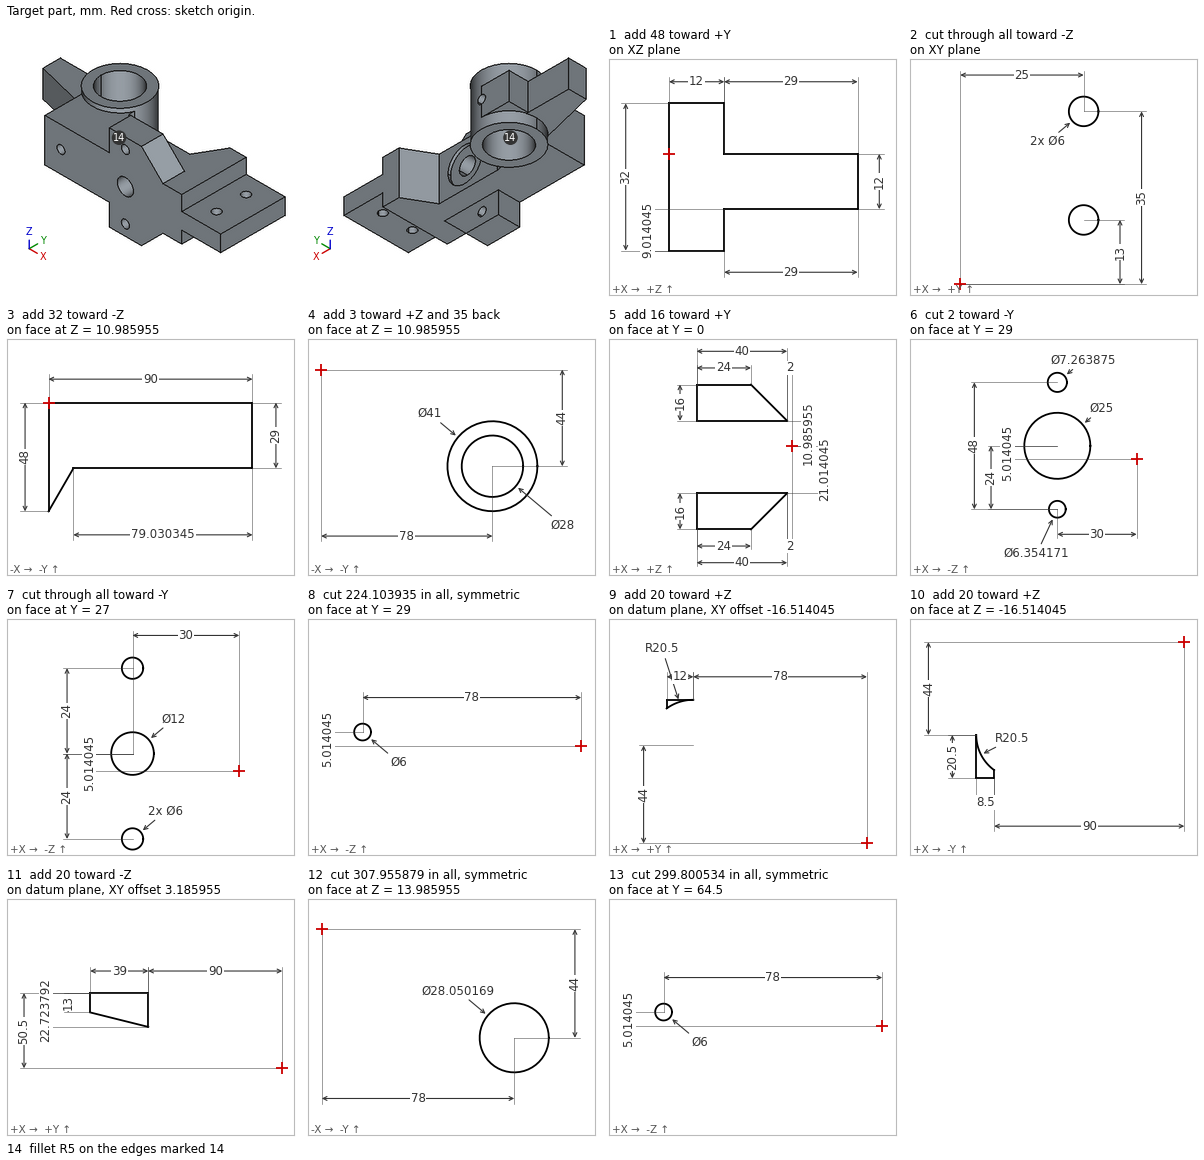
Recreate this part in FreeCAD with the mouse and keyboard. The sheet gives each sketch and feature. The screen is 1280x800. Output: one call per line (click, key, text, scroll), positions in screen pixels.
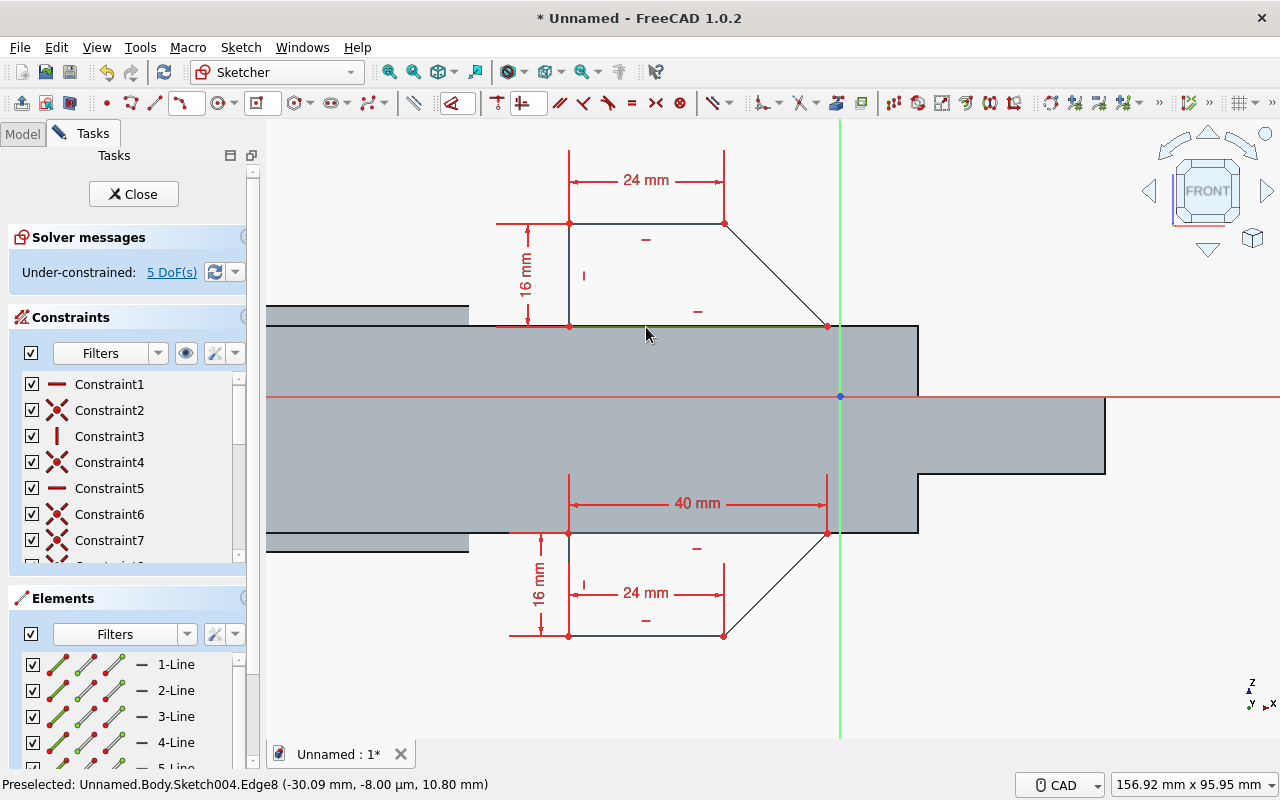
key(l)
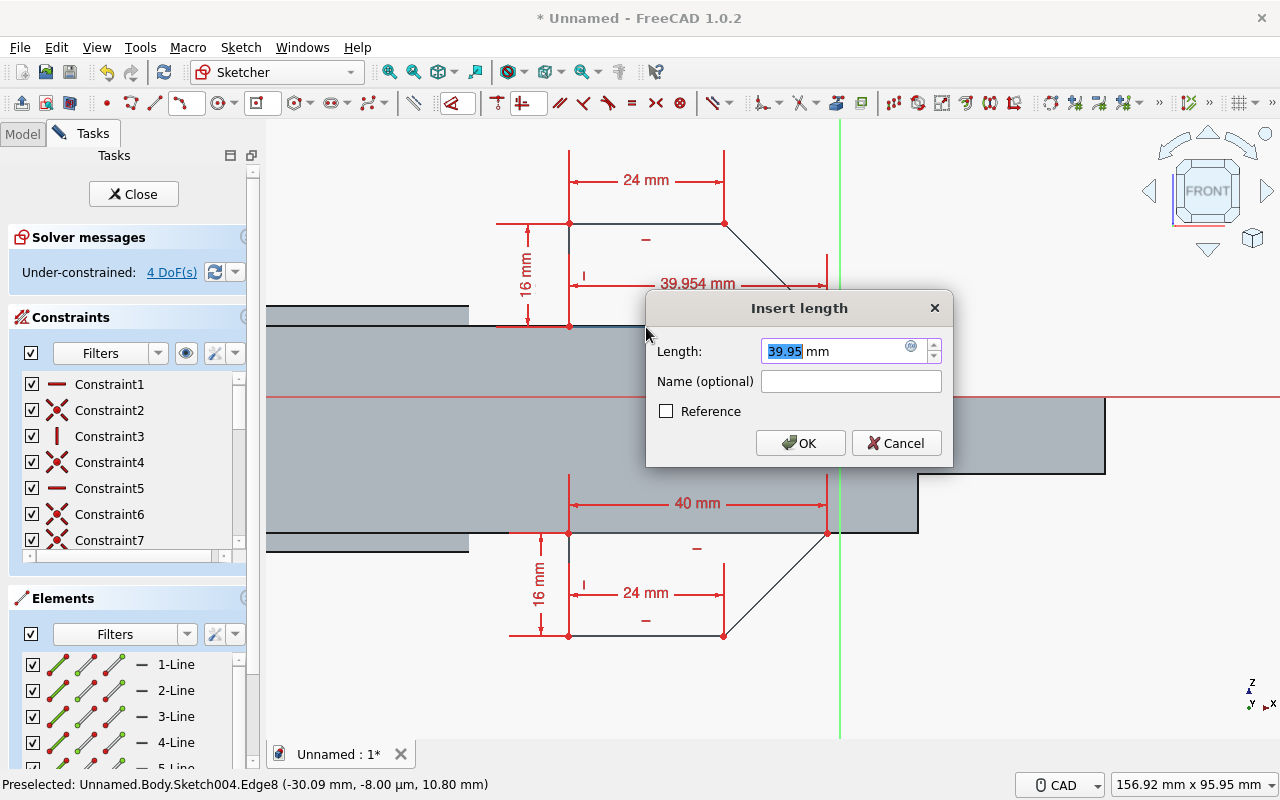
text(40)
key(Return)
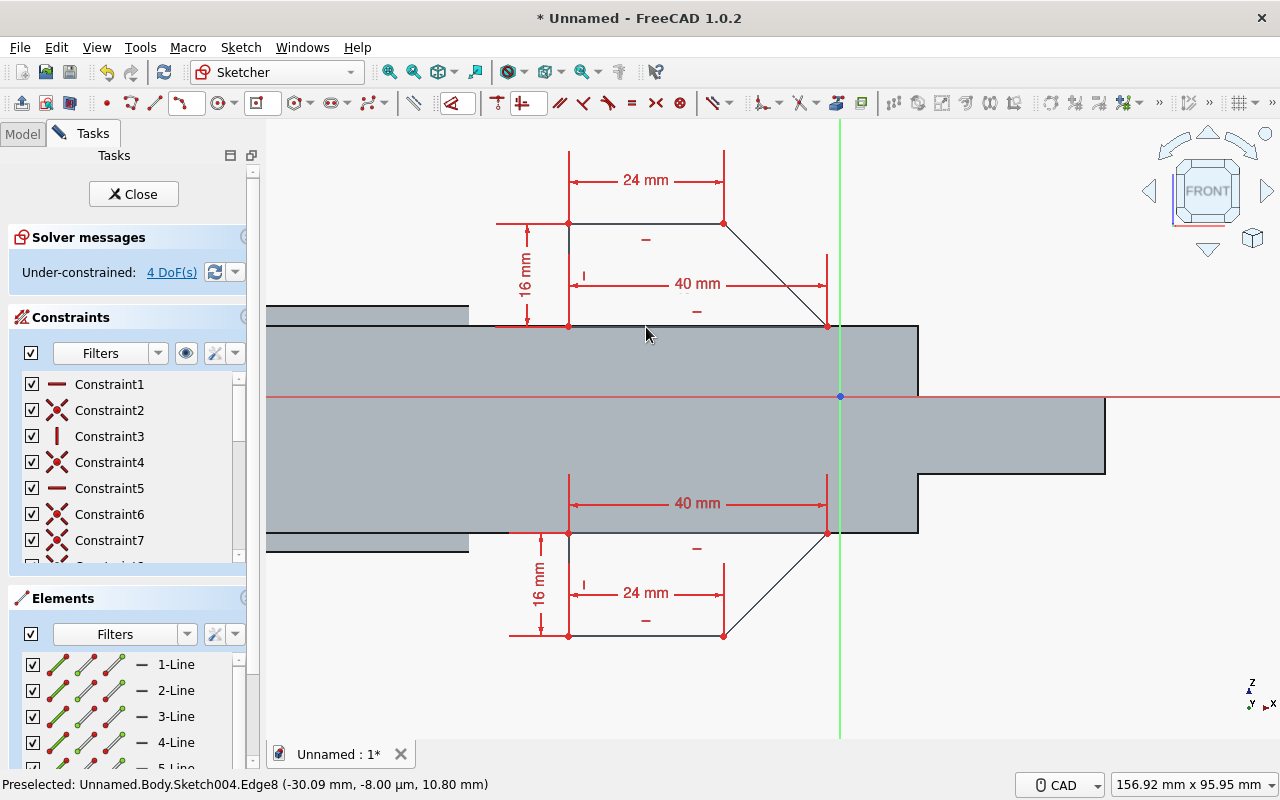
scroll(827, 533, up, 6)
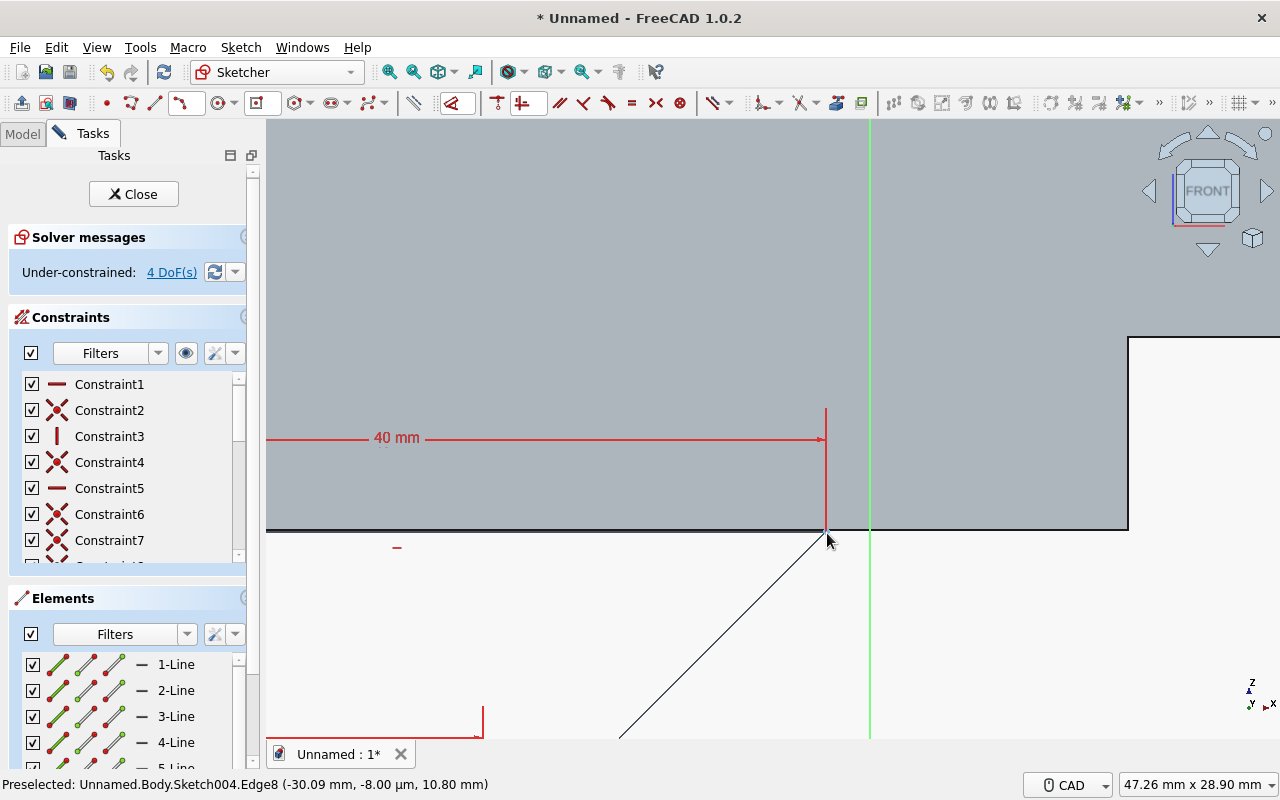
click(826, 532)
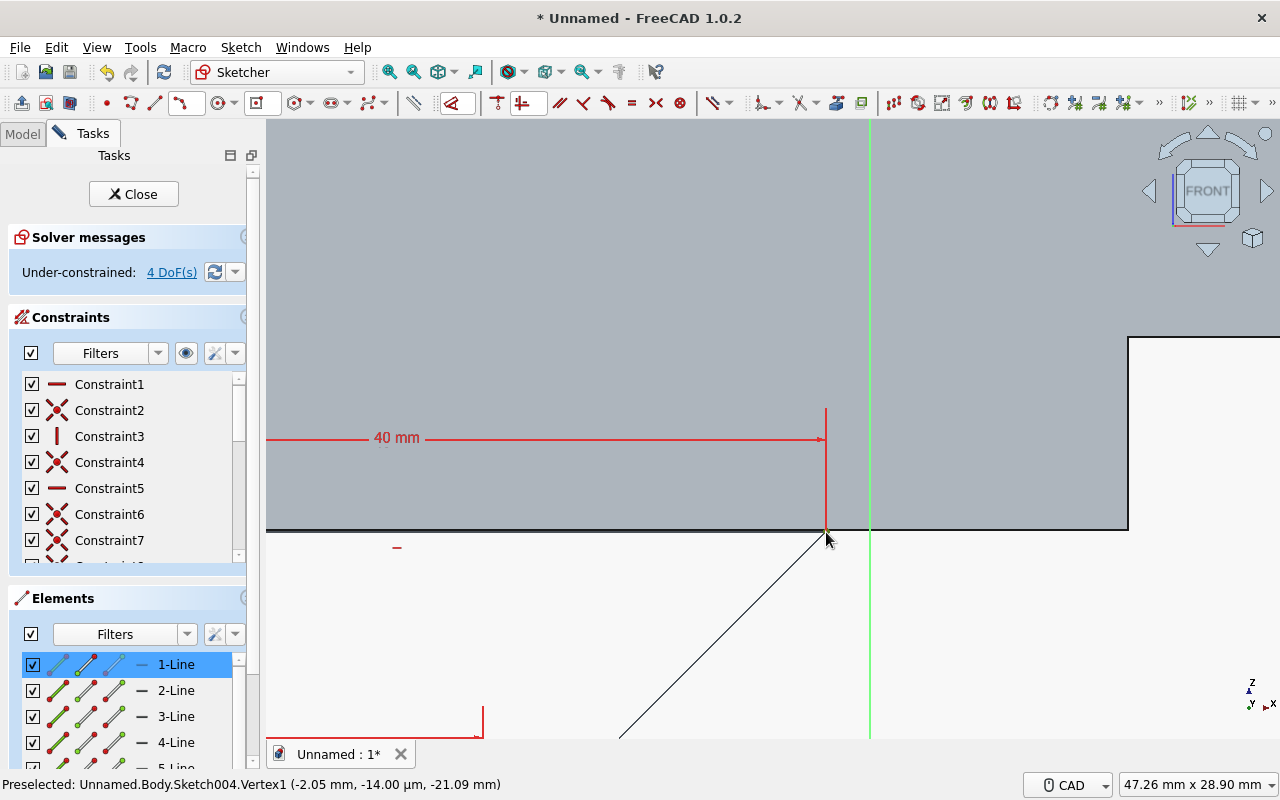
click(470, 104)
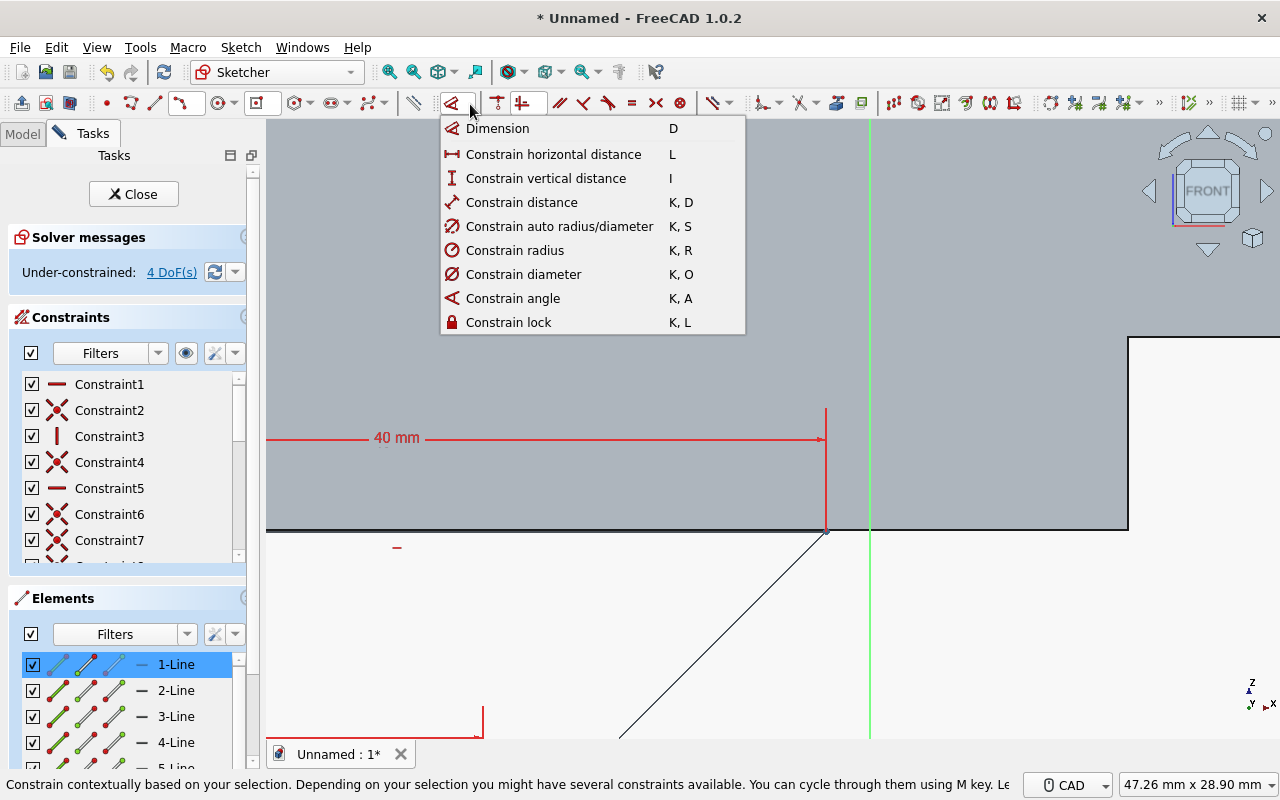
click(593, 154)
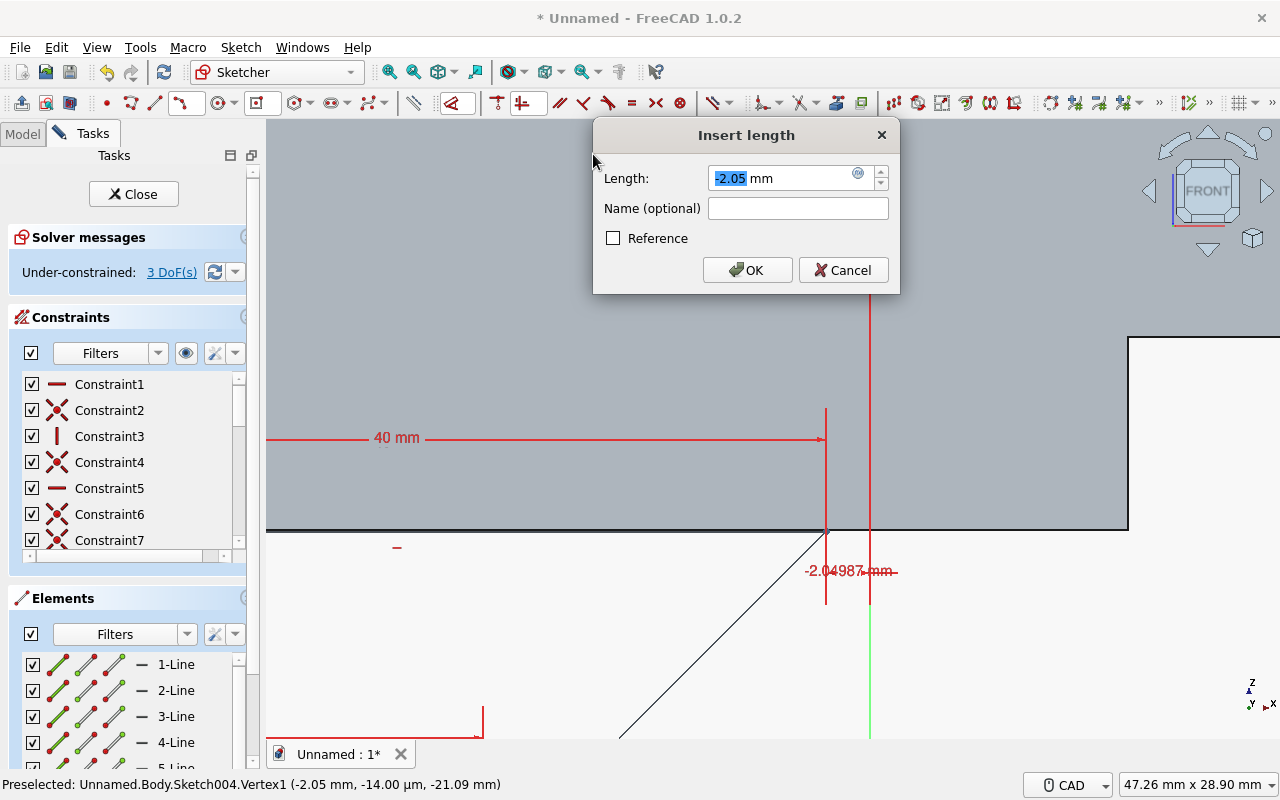
text(-2)
key(Return)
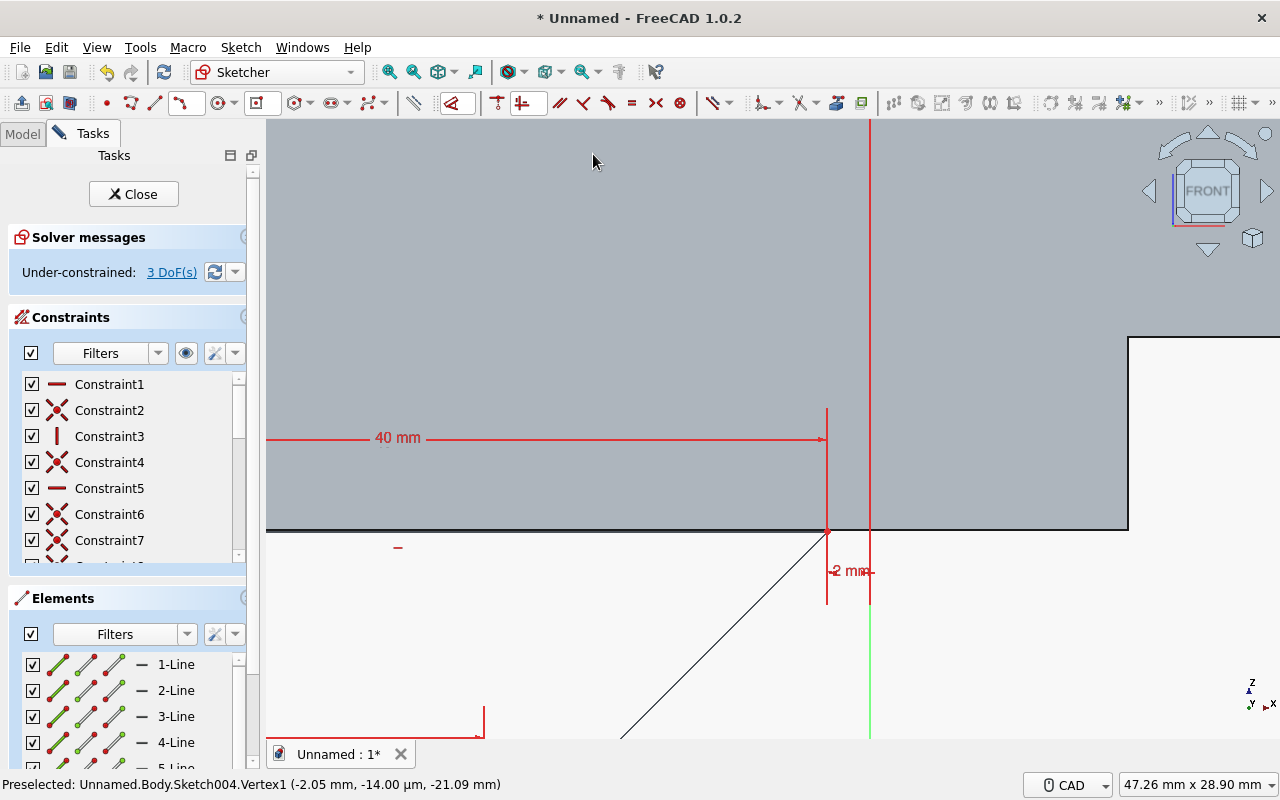
scroll(827, 533, down, 6)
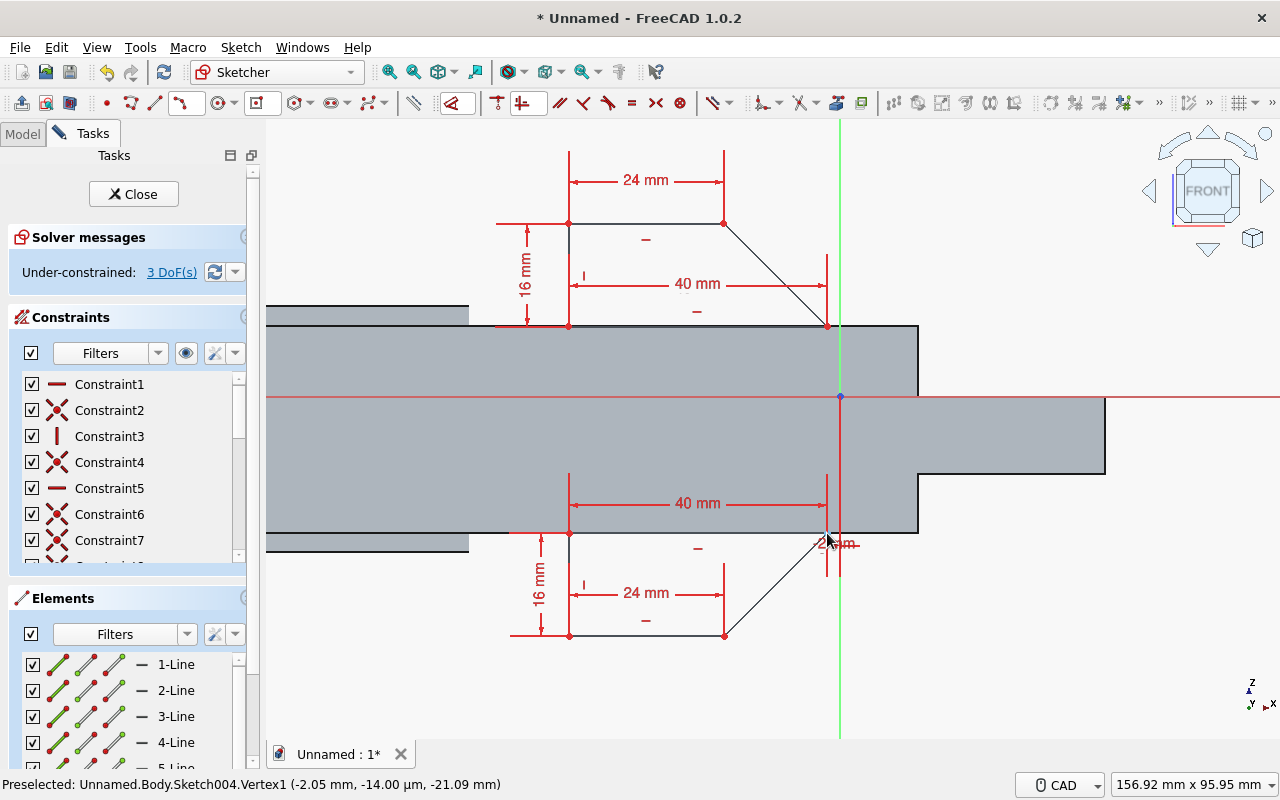
scroll(827, 327, up, 6)